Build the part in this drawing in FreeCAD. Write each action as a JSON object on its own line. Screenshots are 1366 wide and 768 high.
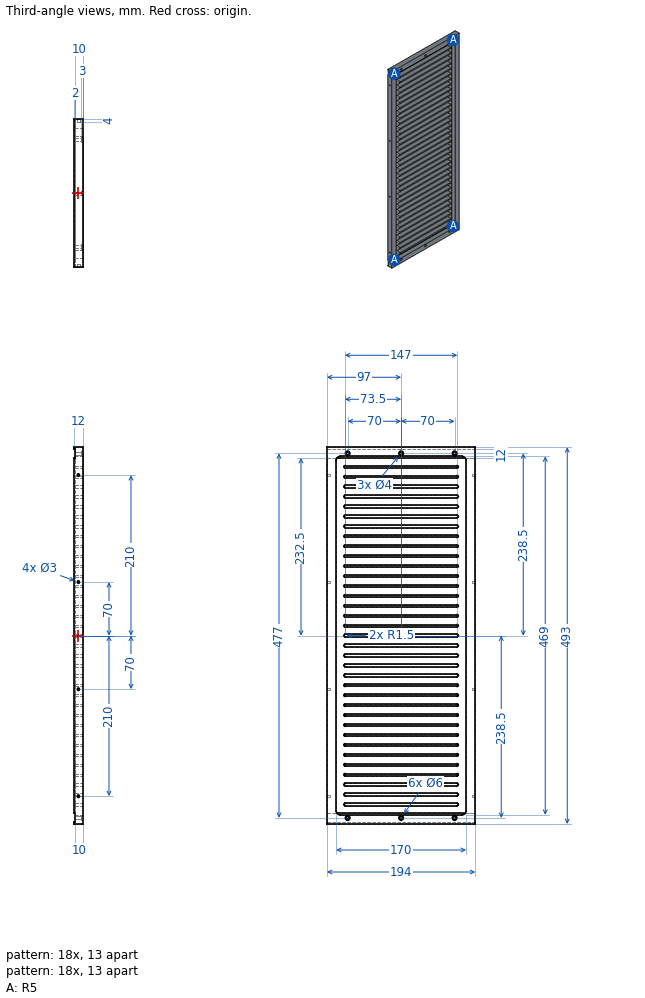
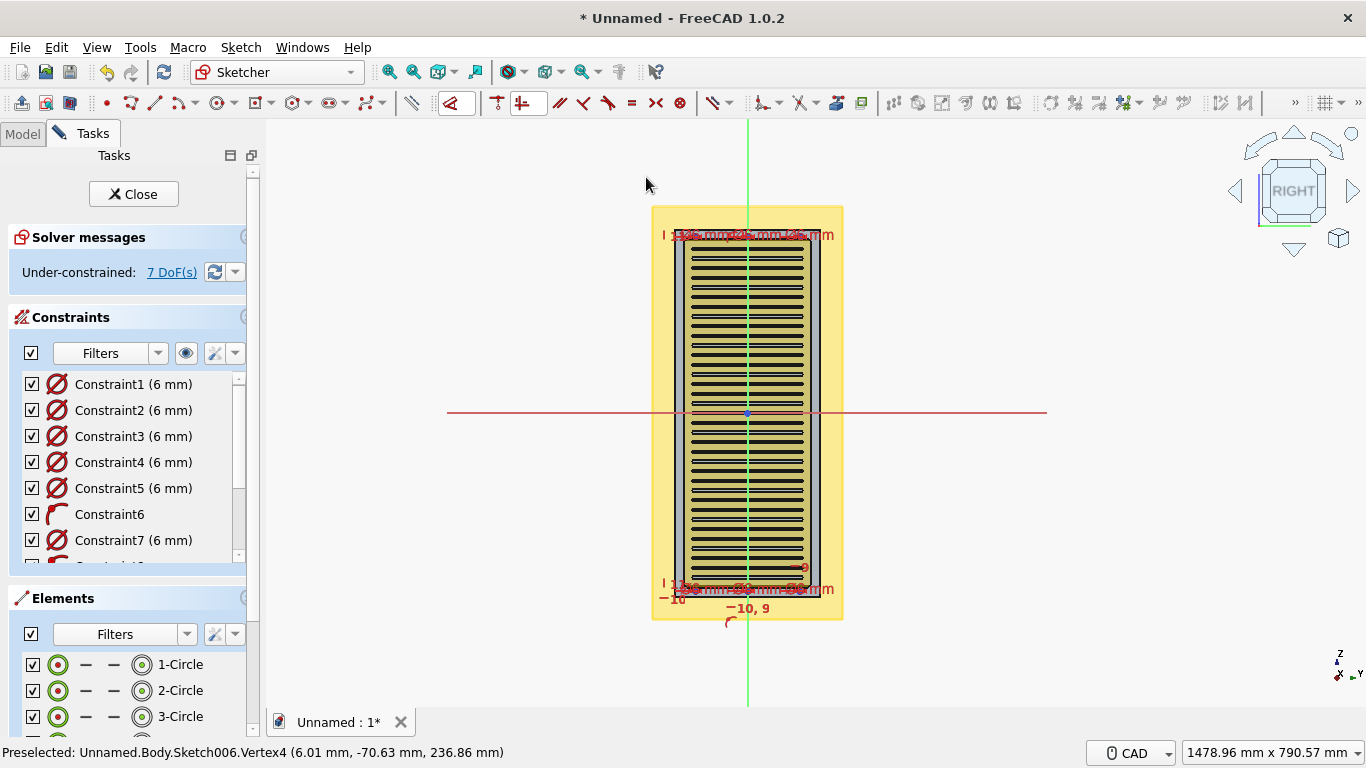
{"action": "left_click", "coordinate": [695, 237]}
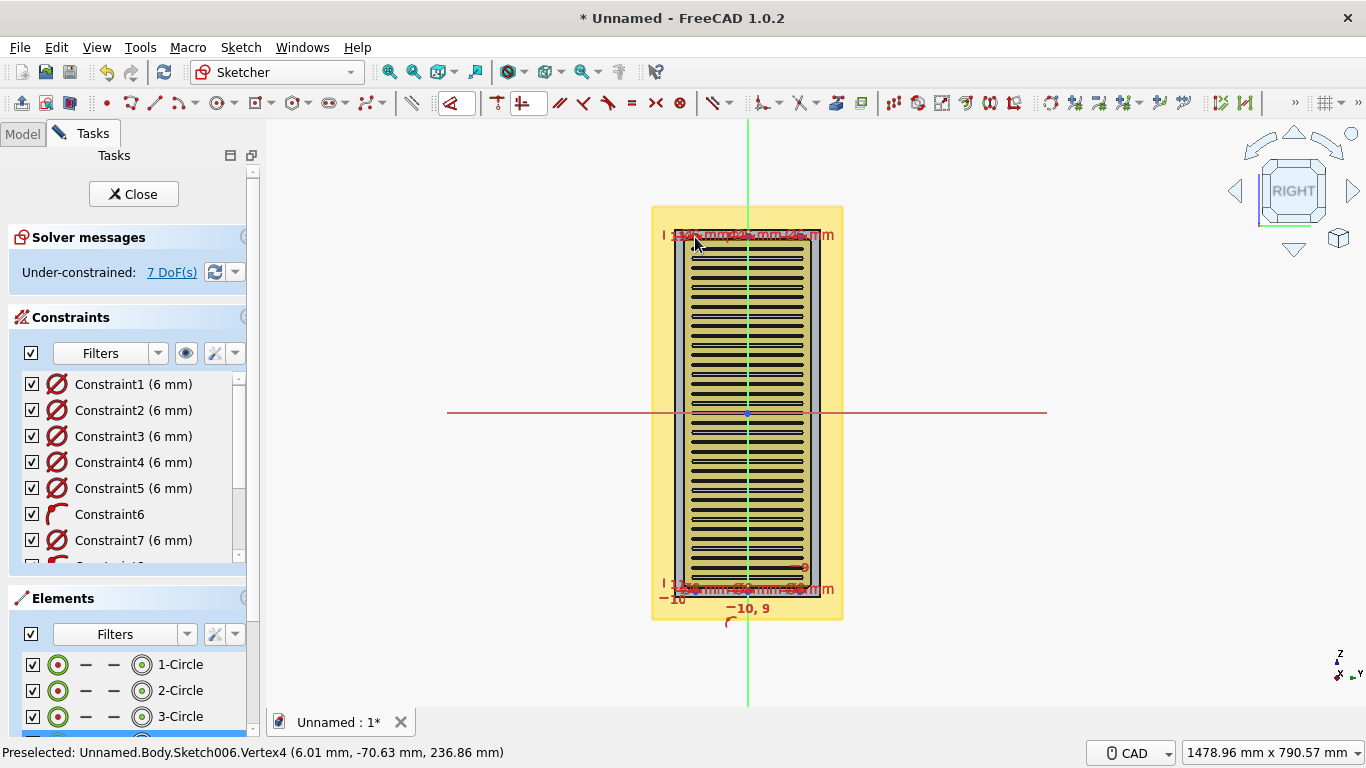
{"action": "left_click", "coordinate": [748, 237]}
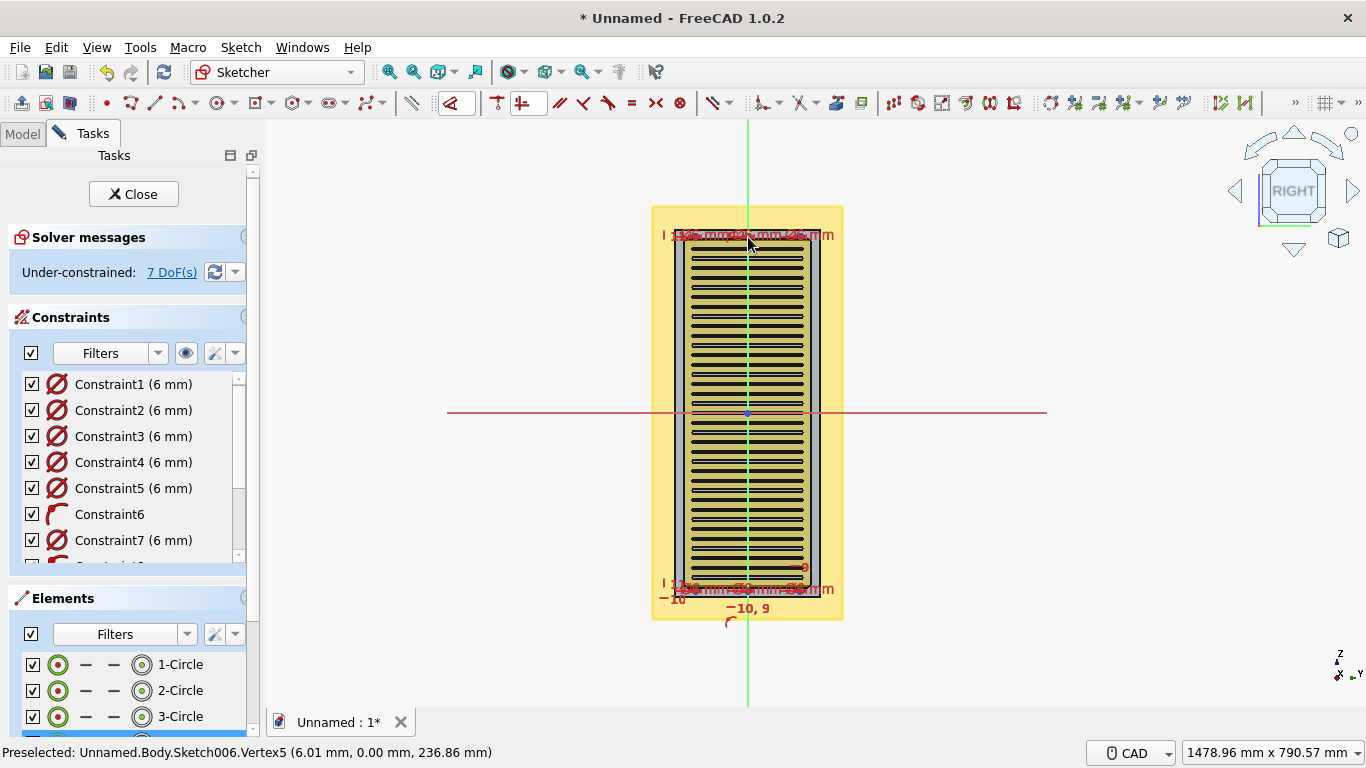
{"action": "left_click", "coordinate": [542, 104]}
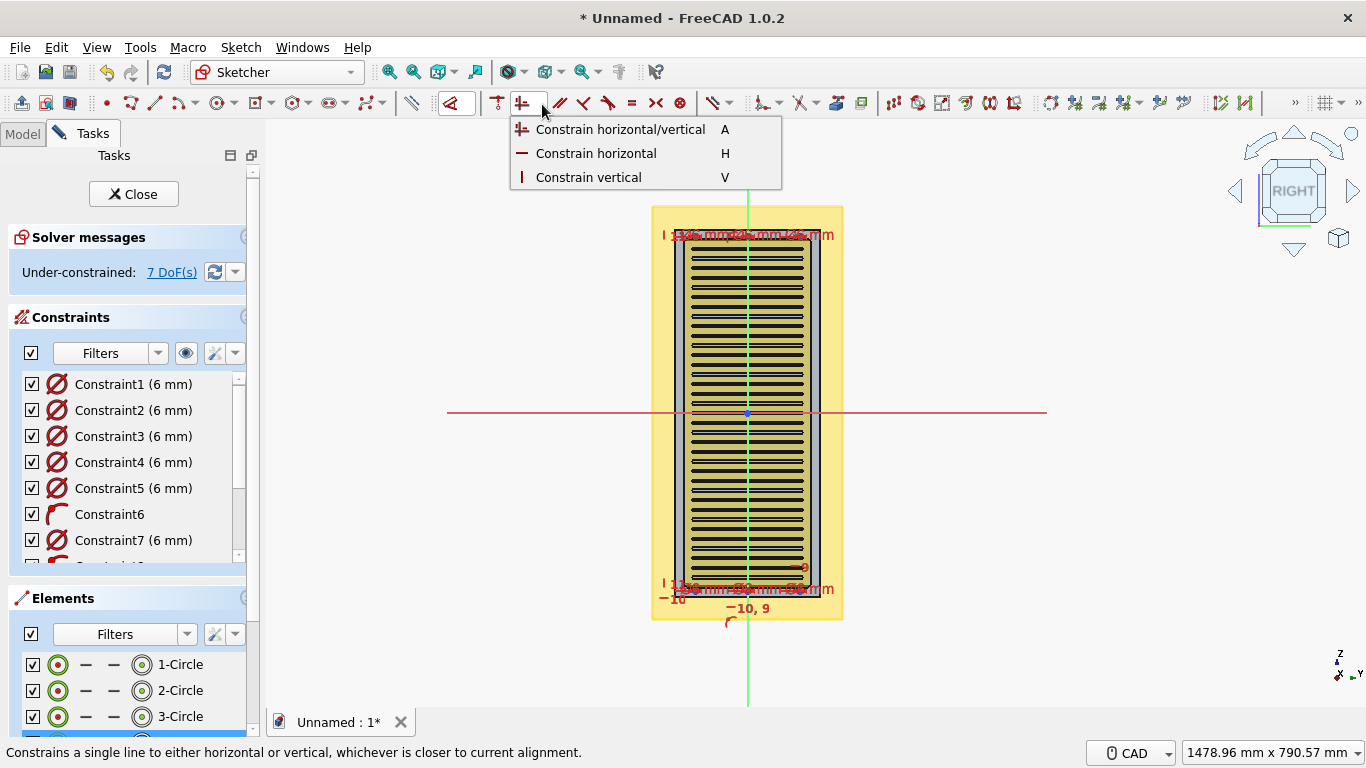
{"action": "left_click", "coordinate": [646, 153]}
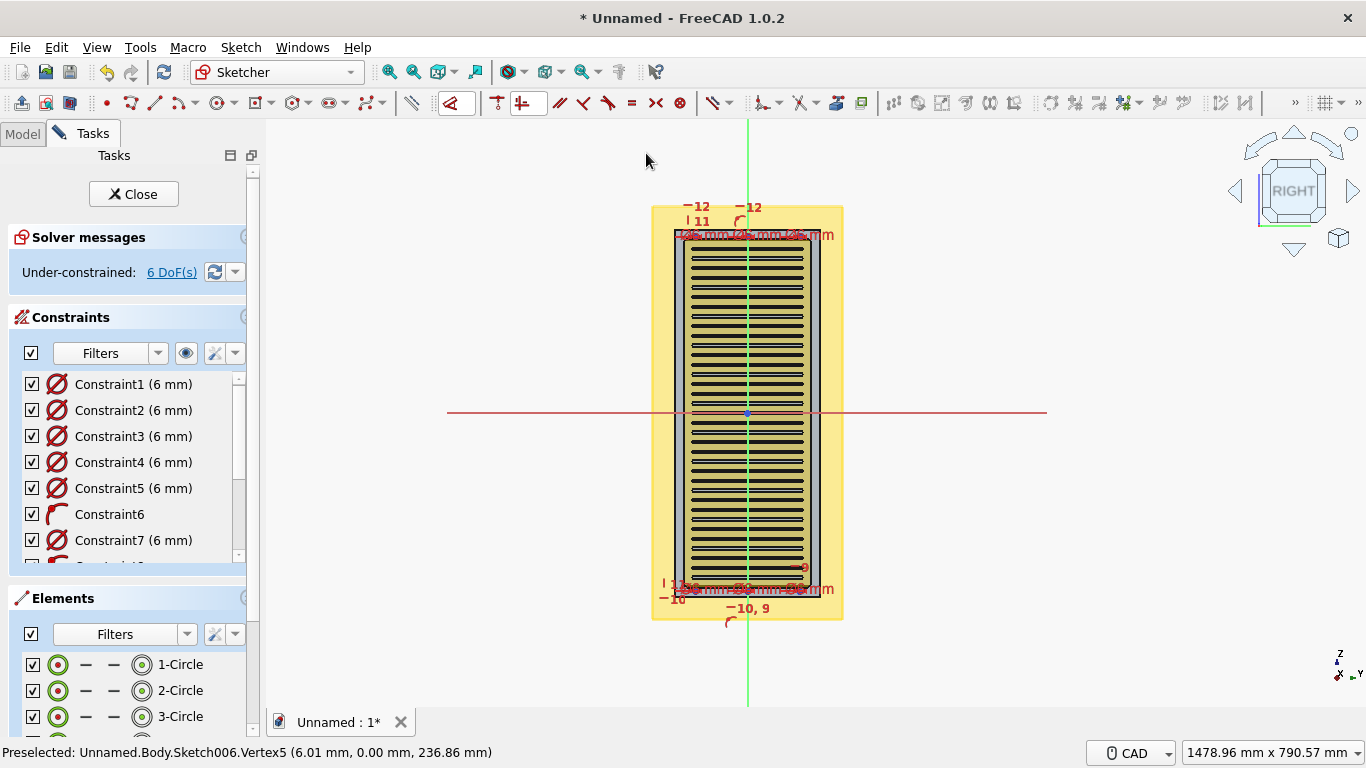
{"action": "left_click", "coordinate": [800, 591]}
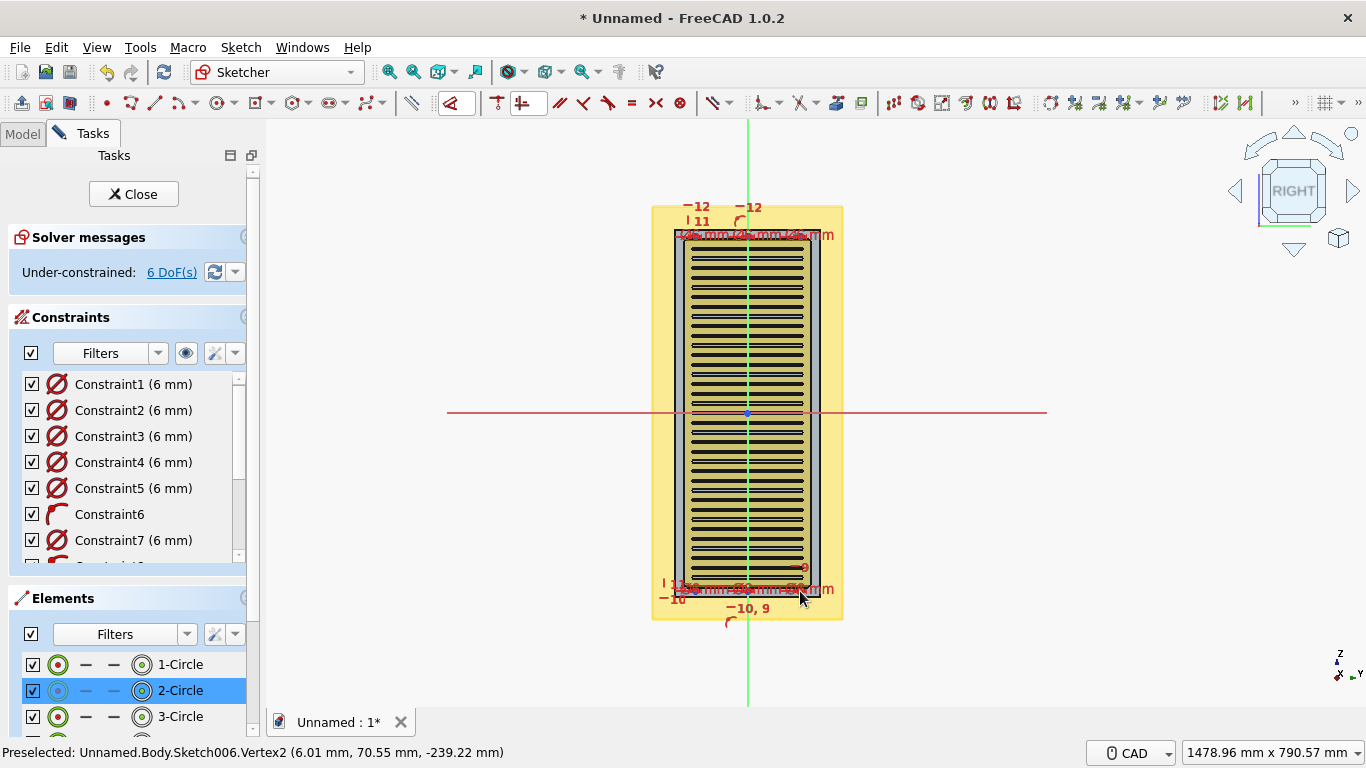
{"action": "left_click", "coordinate": [800, 237]}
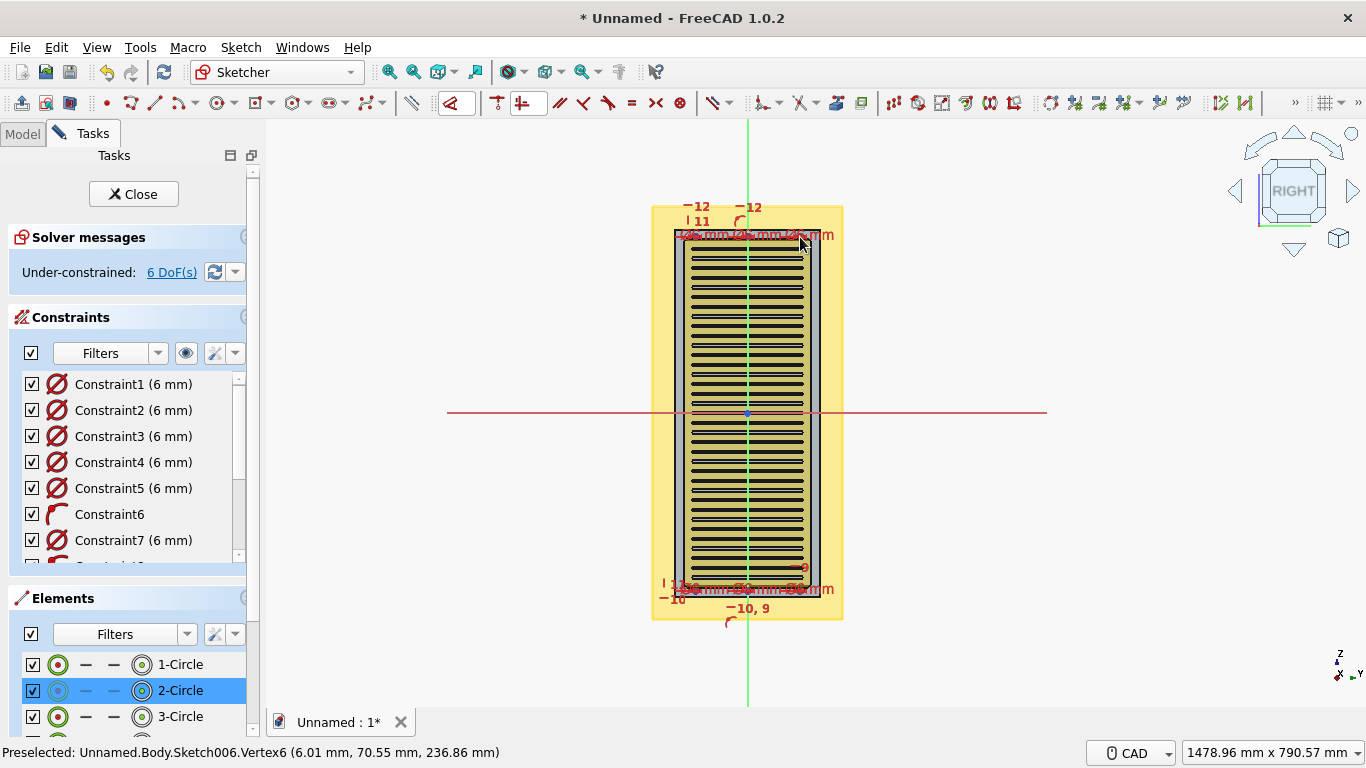
{"action": "left_click", "coordinate": [542, 104]}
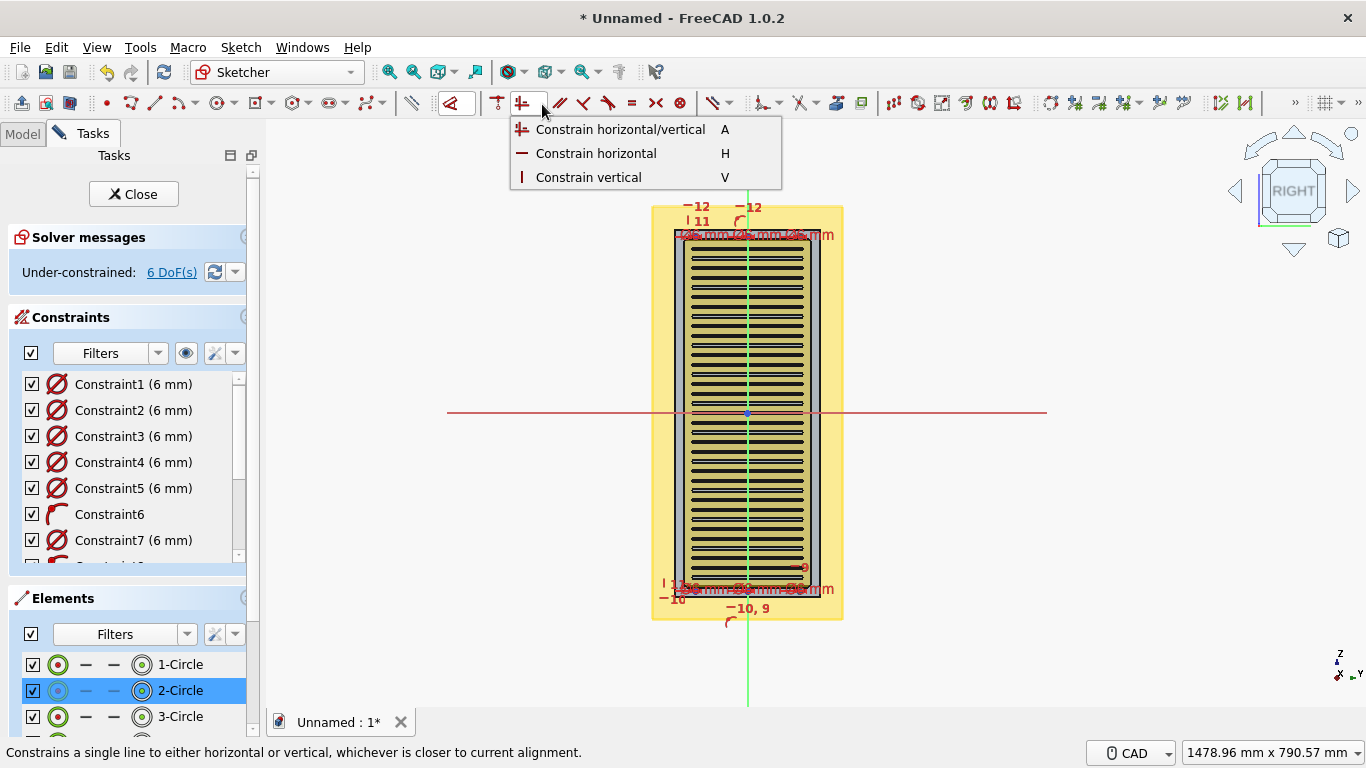
{"action": "left_click", "coordinate": [646, 177]}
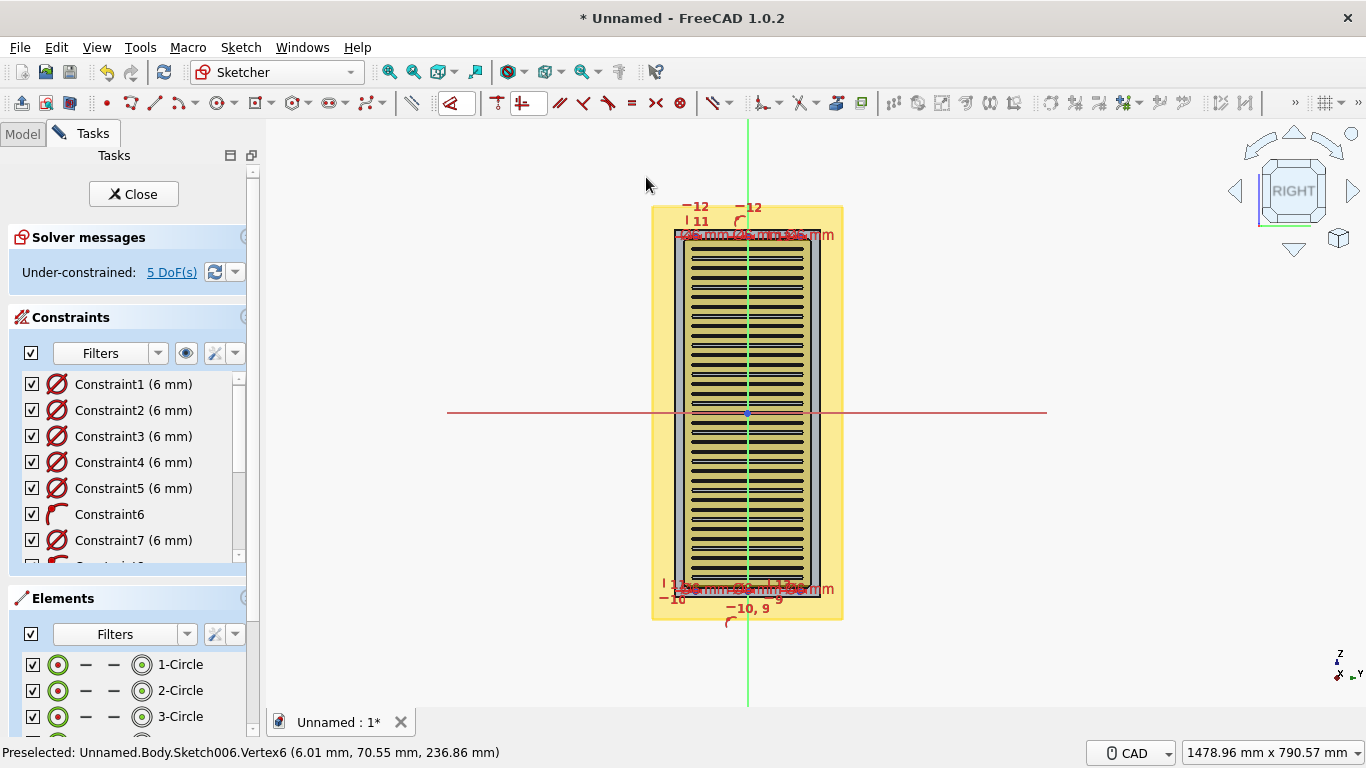
{"action": "left_click", "coordinate": [748, 237]}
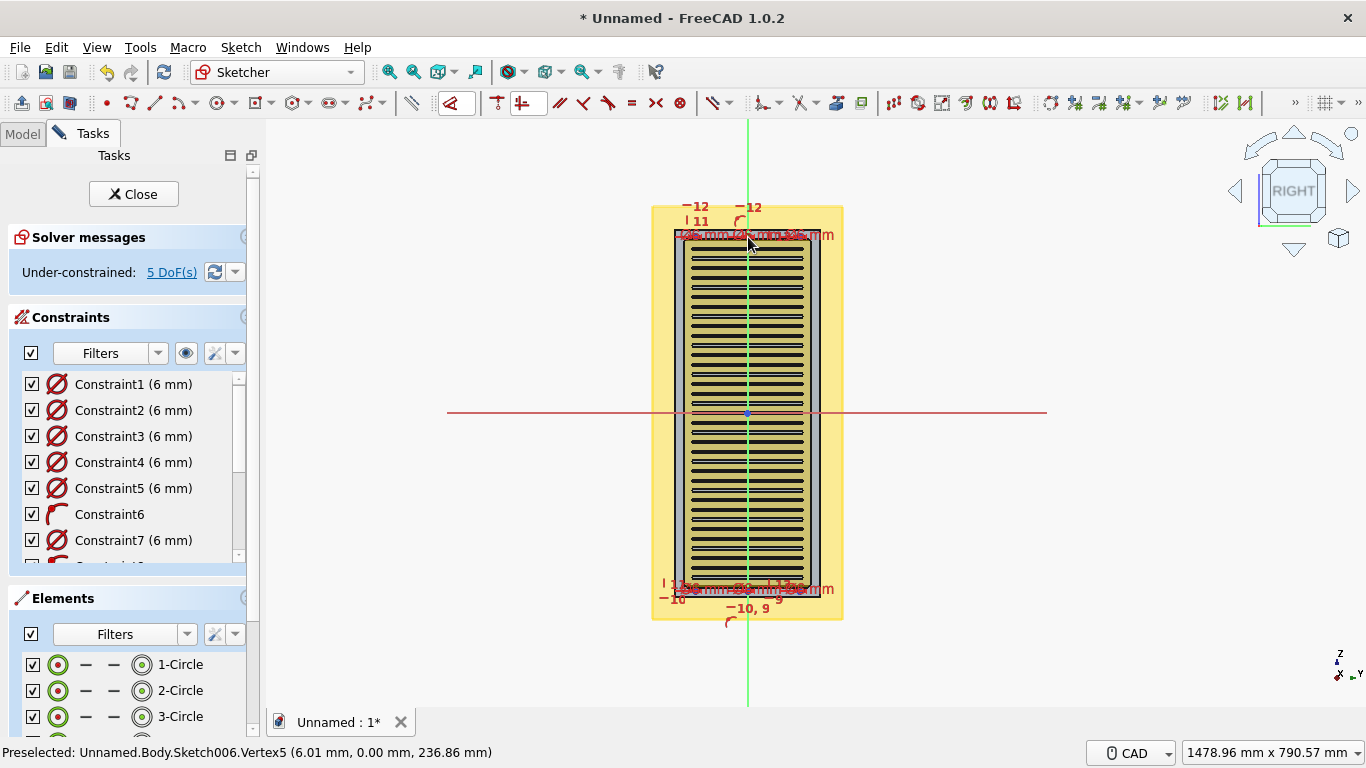
{"action": "left_click", "coordinate": [800, 237]}